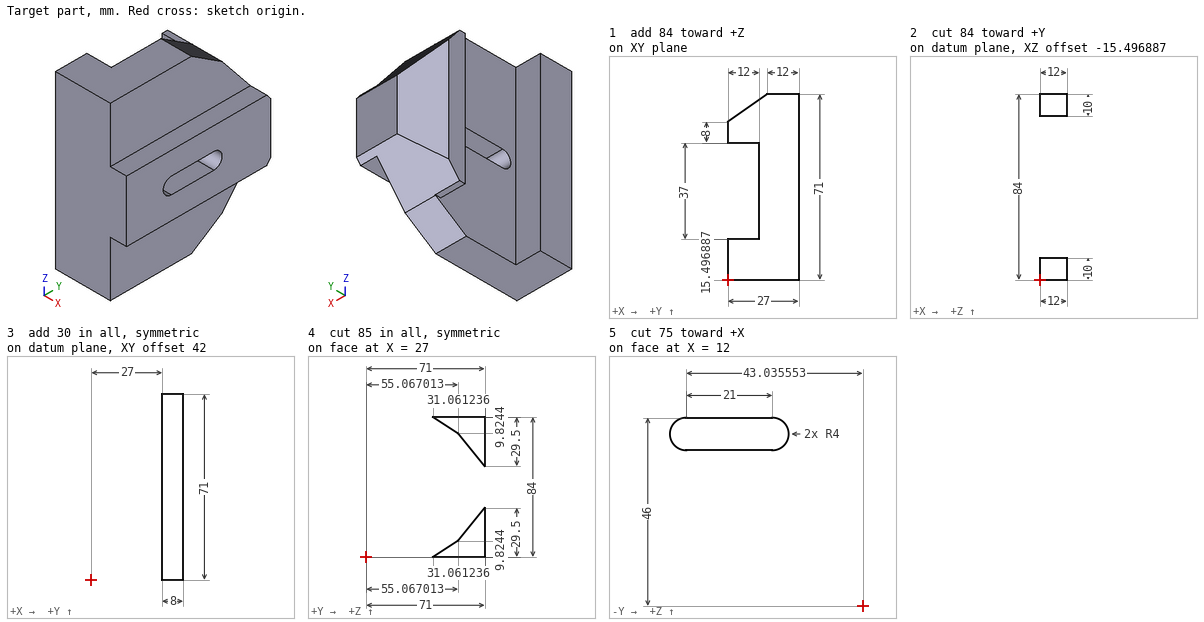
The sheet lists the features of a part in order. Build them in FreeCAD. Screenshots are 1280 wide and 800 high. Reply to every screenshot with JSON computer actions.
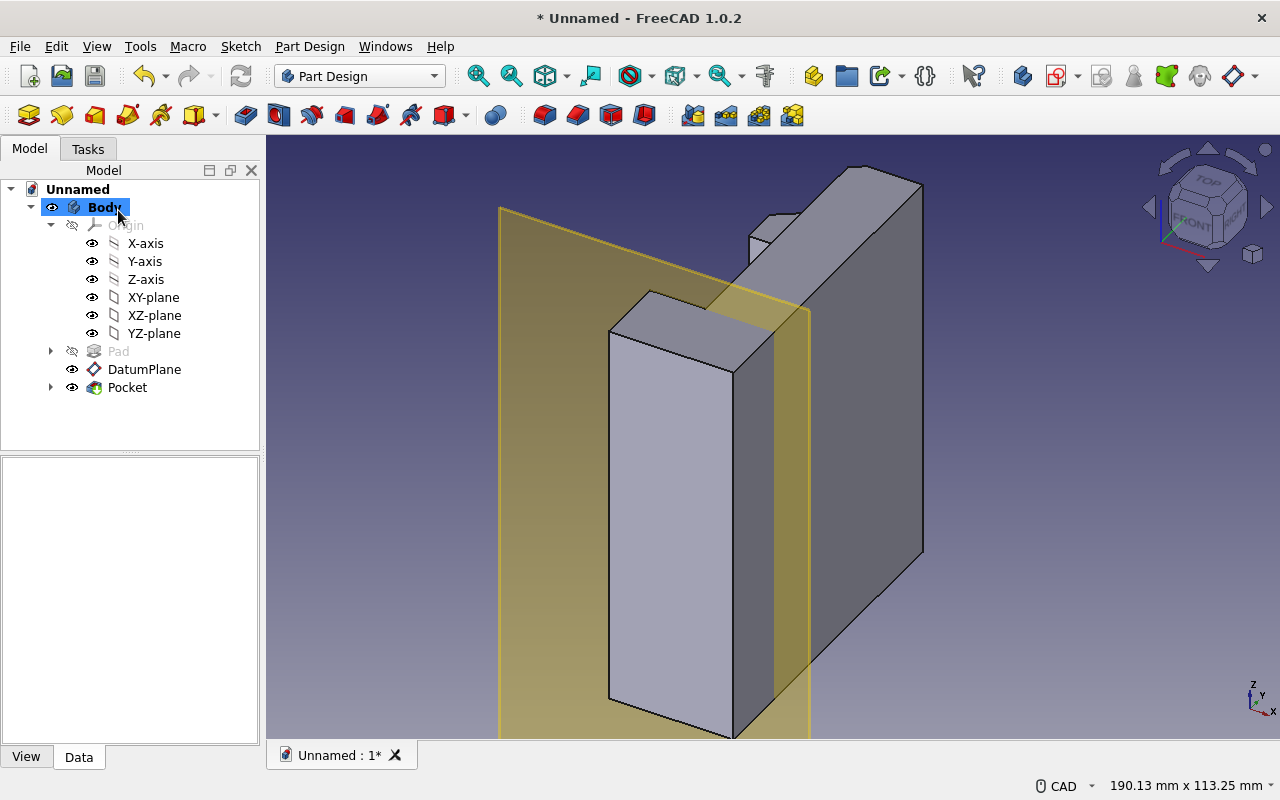
{"action": "left_click", "coordinate": [117, 369]}
{"action": "key", "text": "space"}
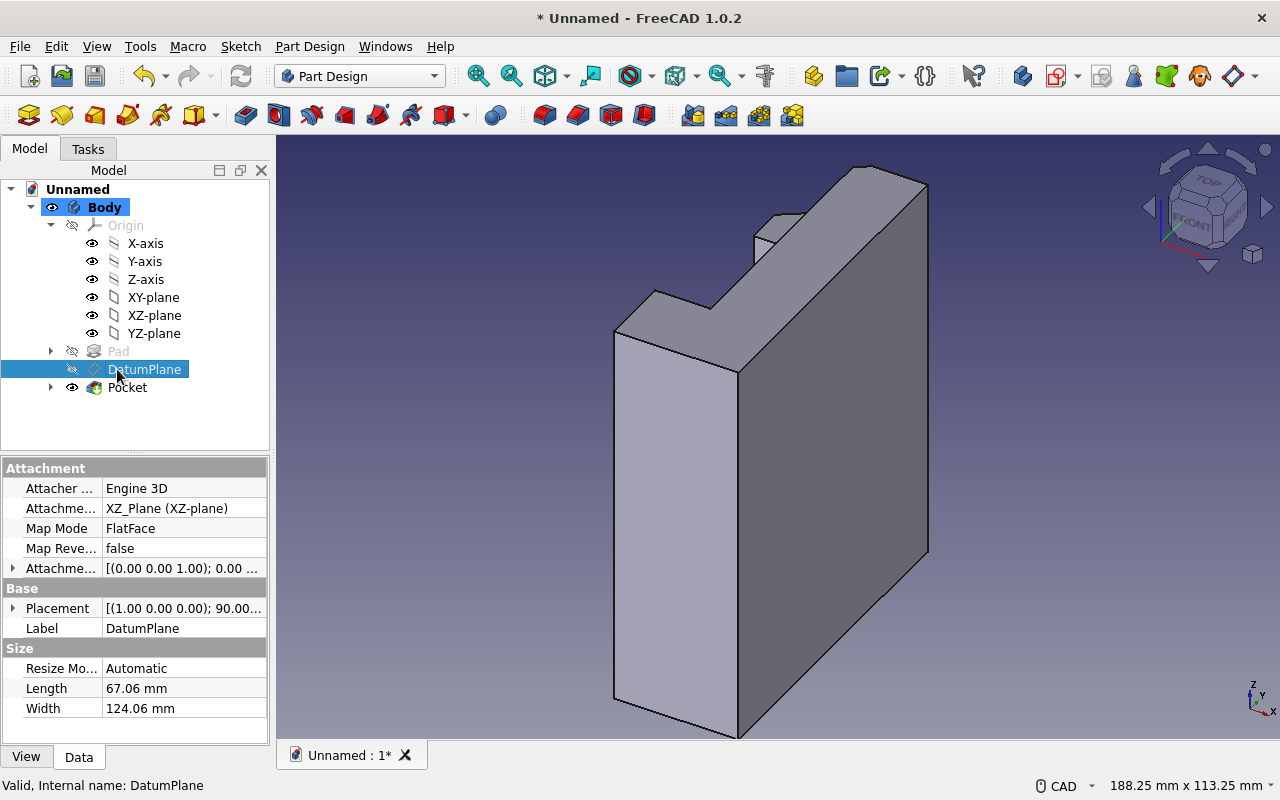
{"action": "left_click", "coordinate": [137, 297]}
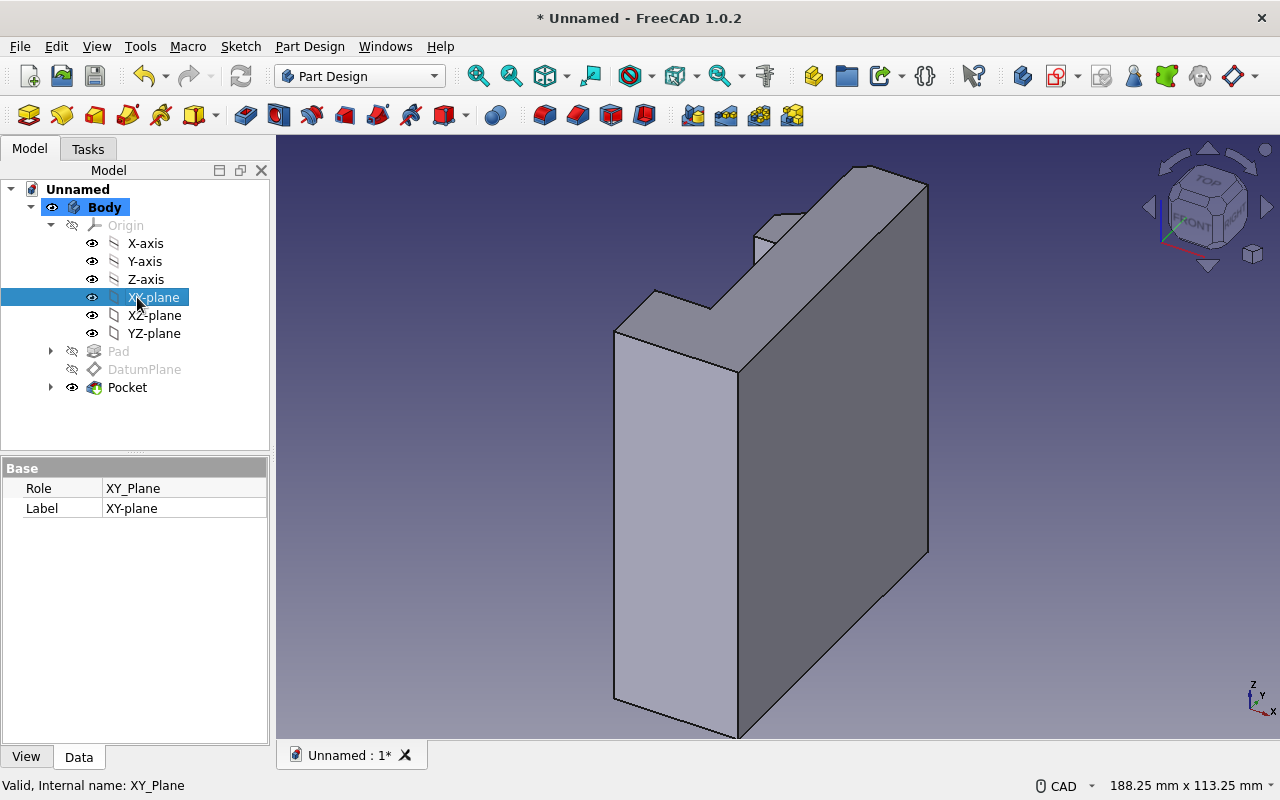
{"action": "left_click", "coordinate": [1232, 76]}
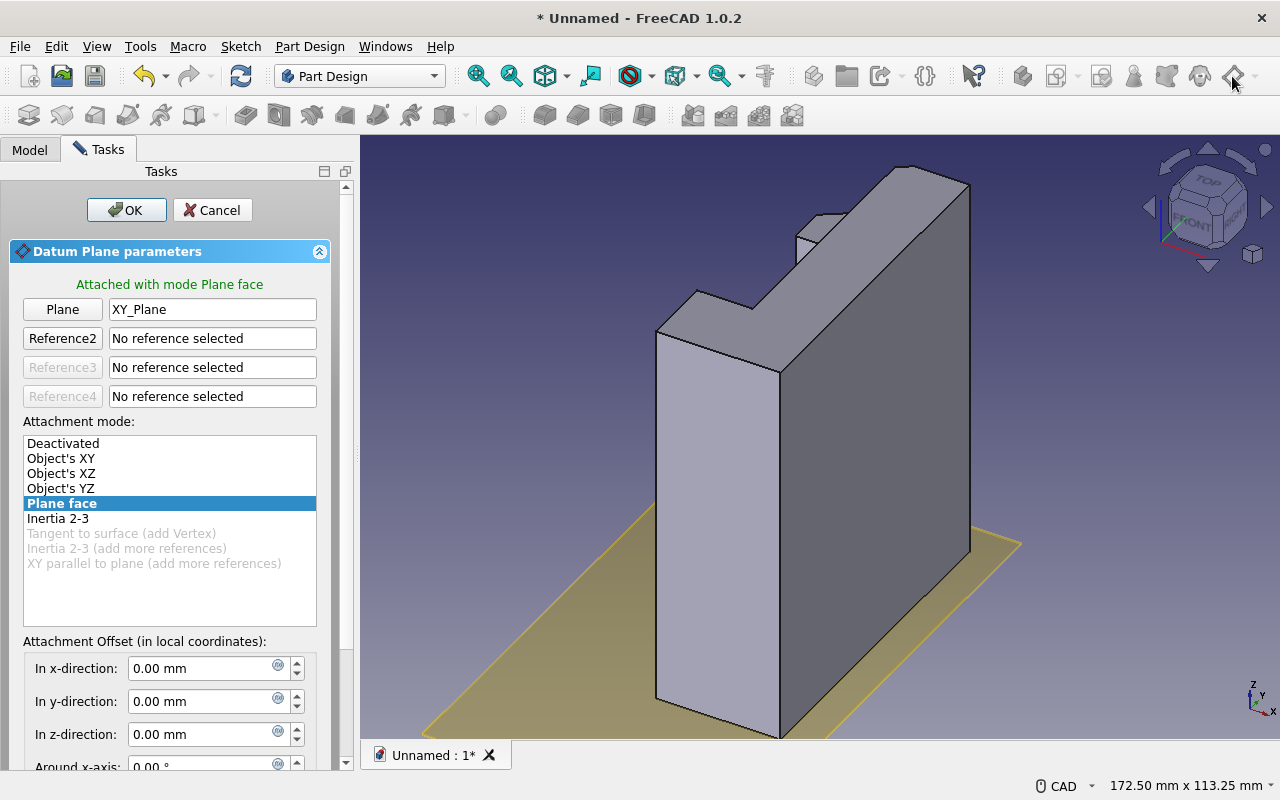
{"action": "triple_click", "coordinate": [210, 734]}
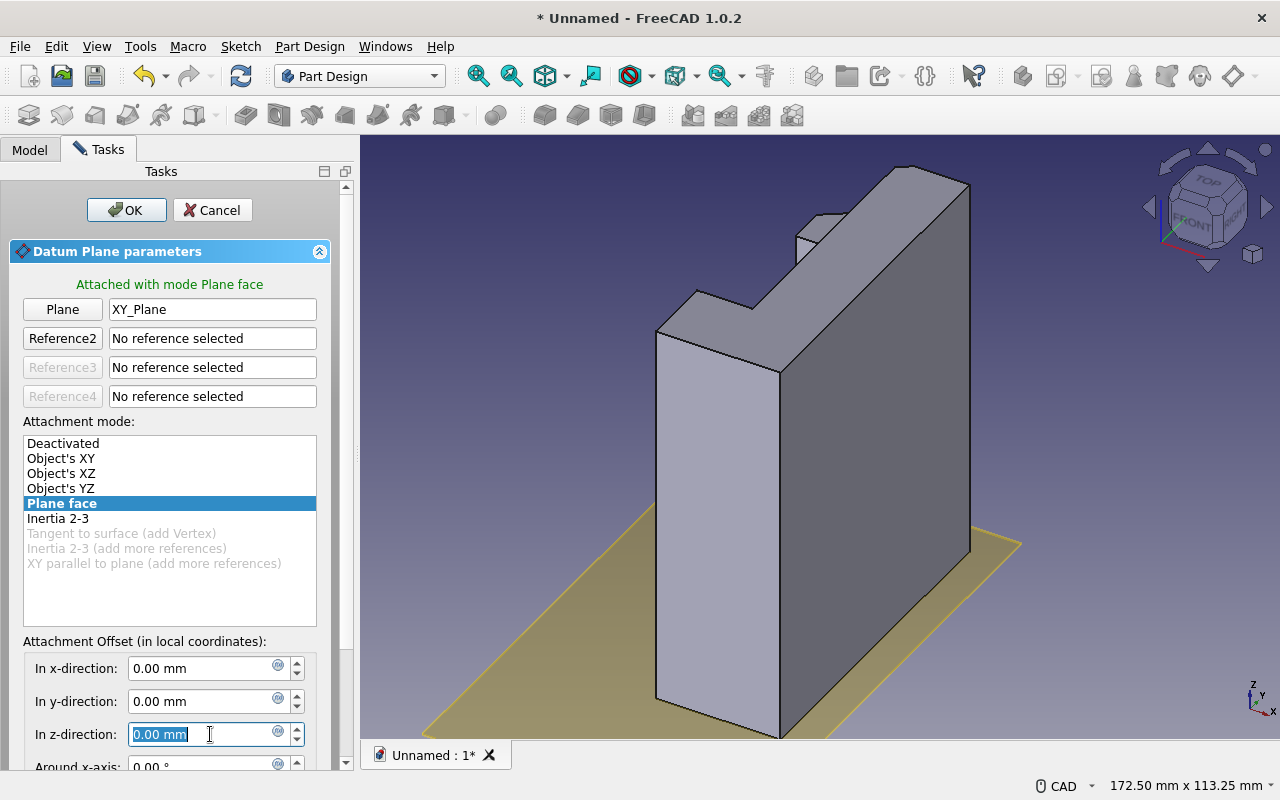
{"action": "type", "text": "42"}
{"action": "key", "text": "Tab"}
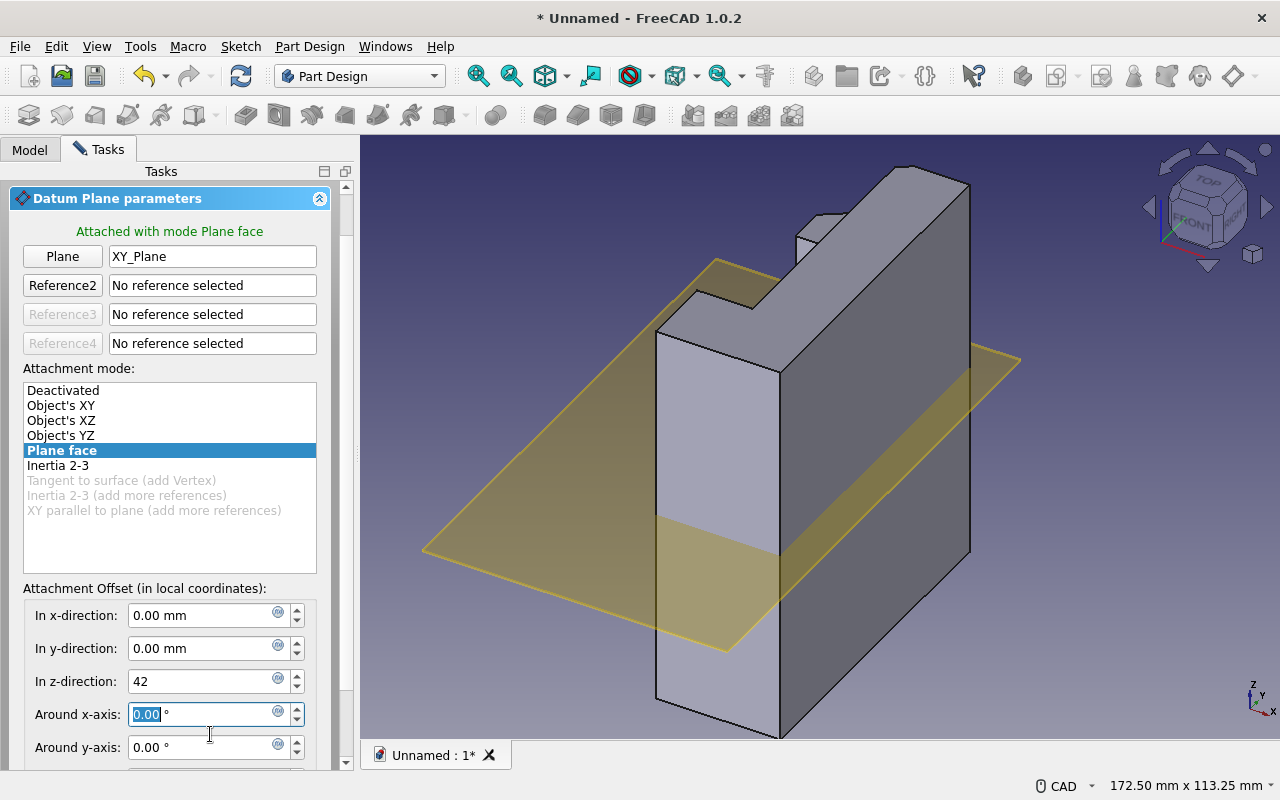
{"action": "scroll", "coordinate": [346, 476], "scroll_direction": "up", "scroll_amount": 2}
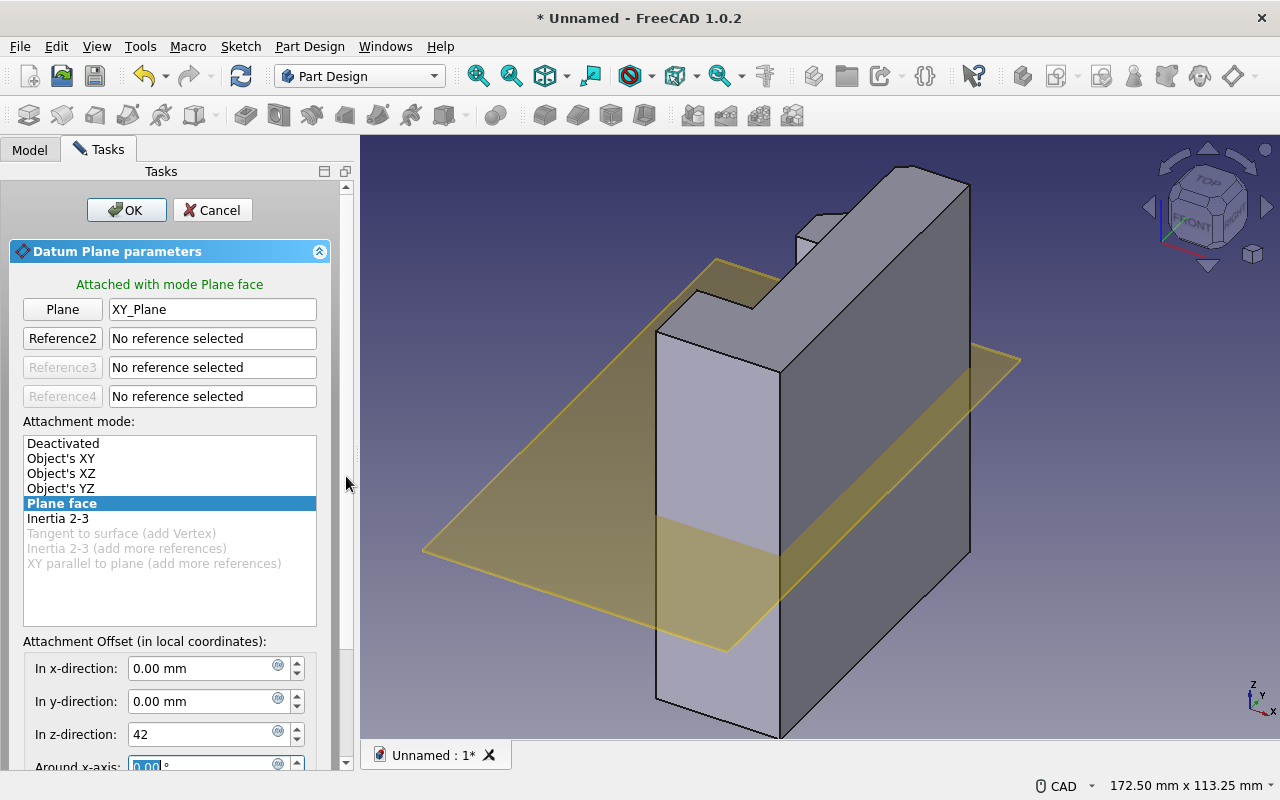
{"action": "left_click", "coordinate": [127, 210]}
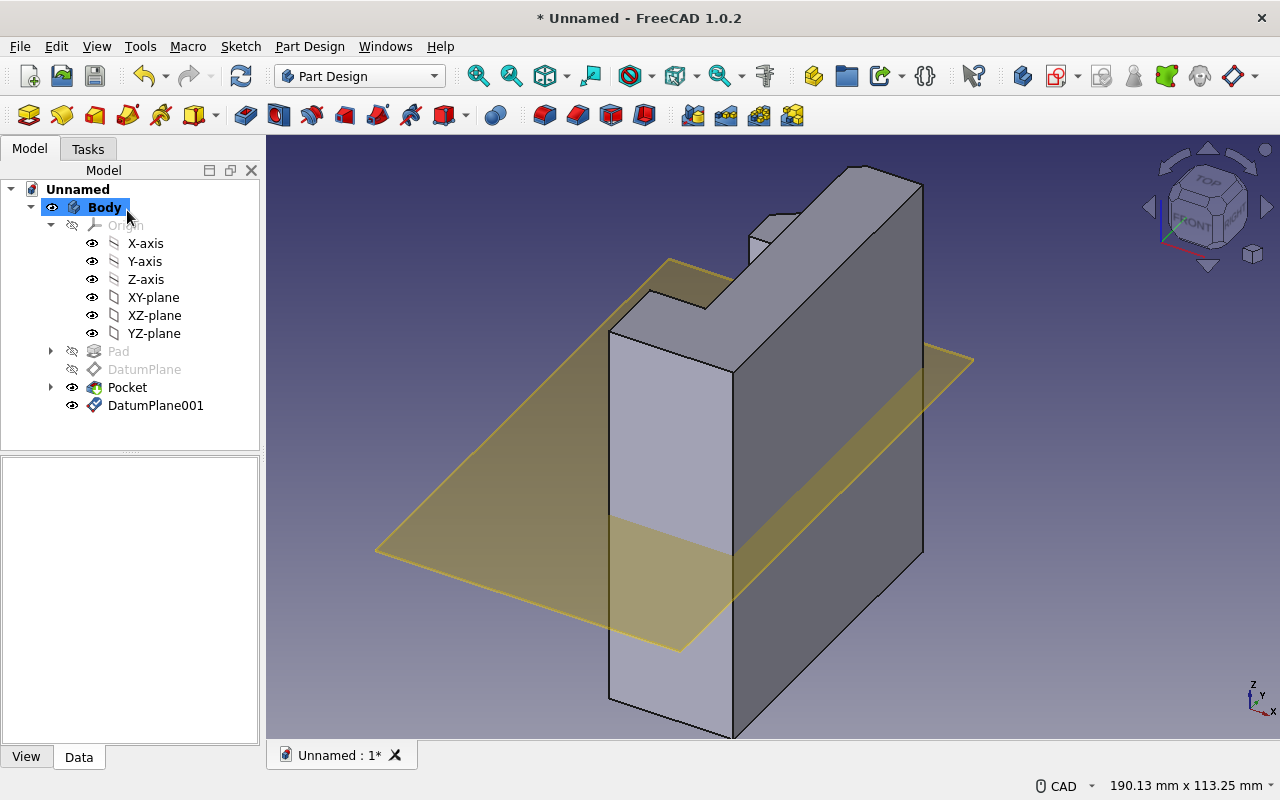
{"action": "left_click", "coordinate": [117, 405]}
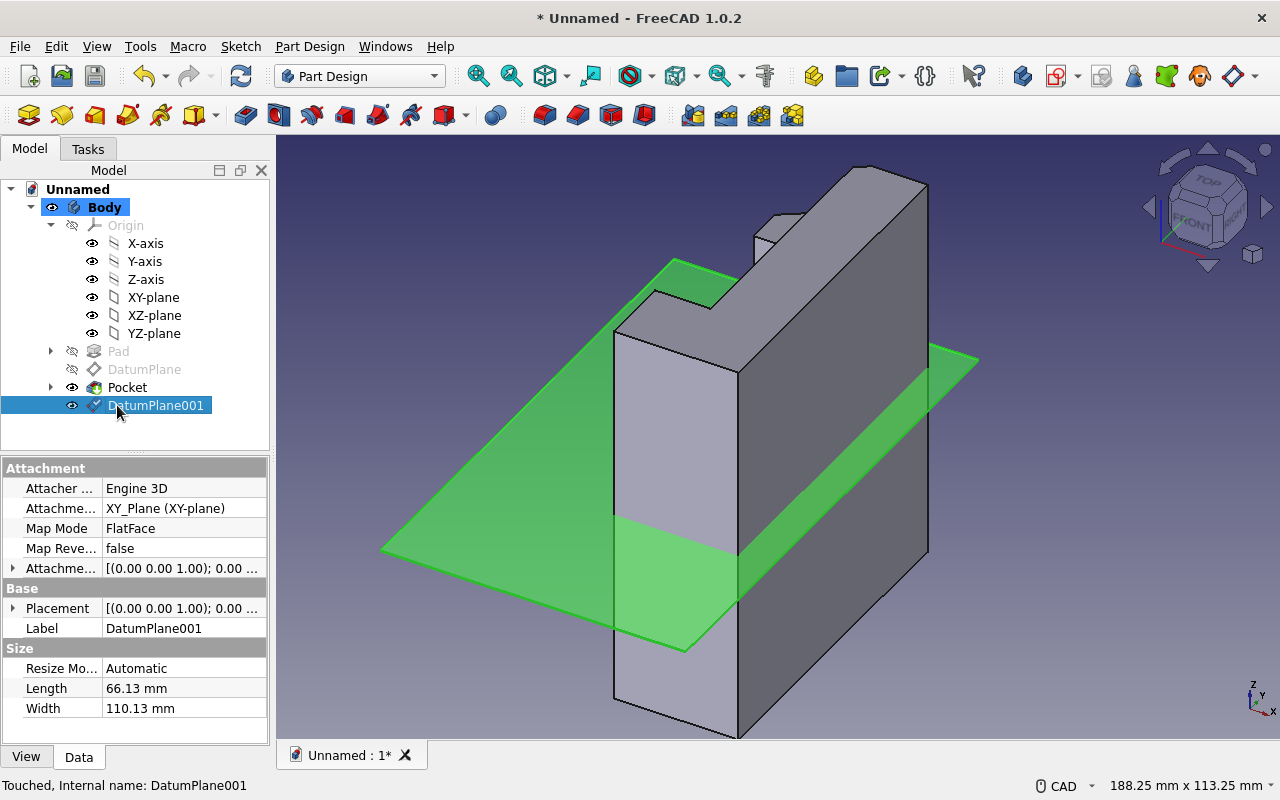
{"action": "left_click", "coordinate": [1056, 76]}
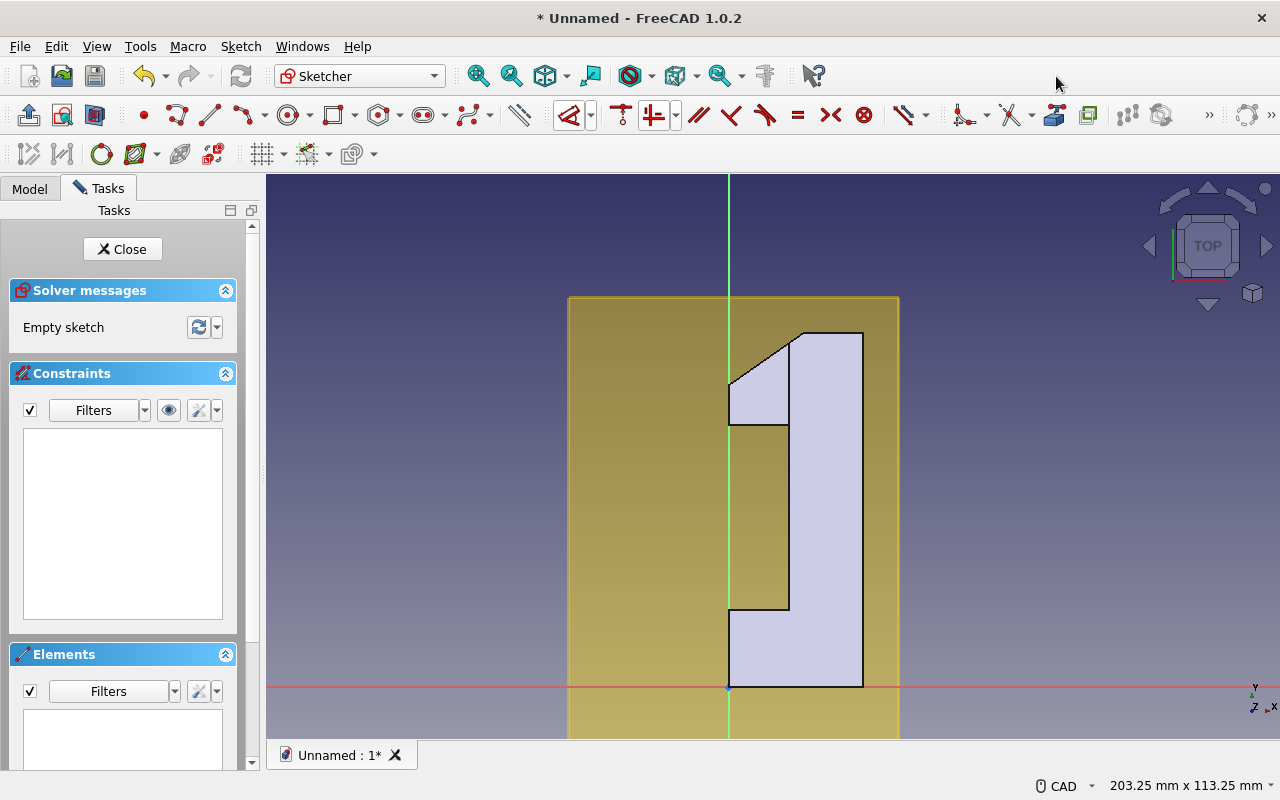
{"action": "left_click", "coordinate": [95, 116]}